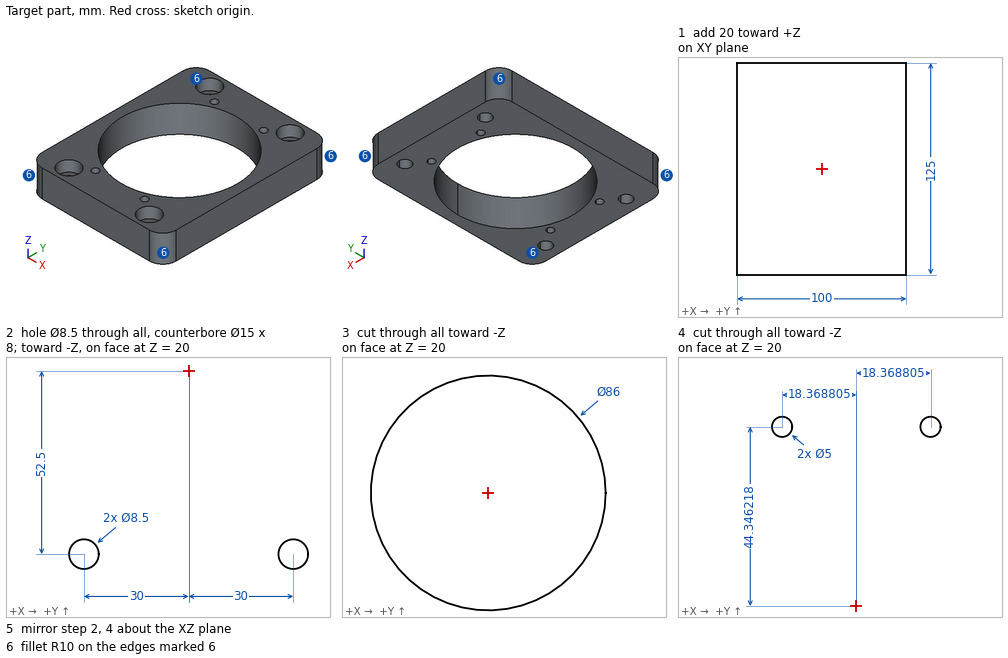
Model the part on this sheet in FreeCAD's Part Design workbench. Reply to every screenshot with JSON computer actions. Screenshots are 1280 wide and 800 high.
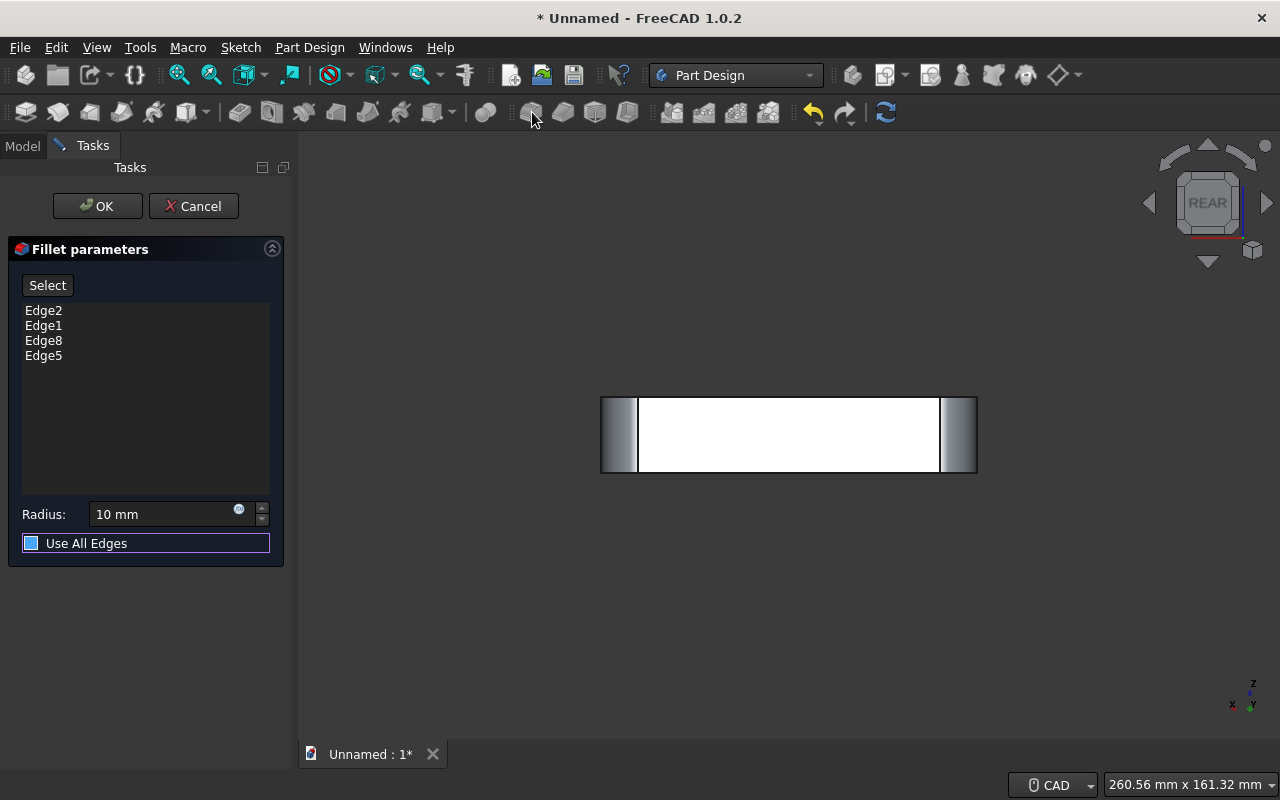
{"action": "left_click", "coordinate": [98, 206]}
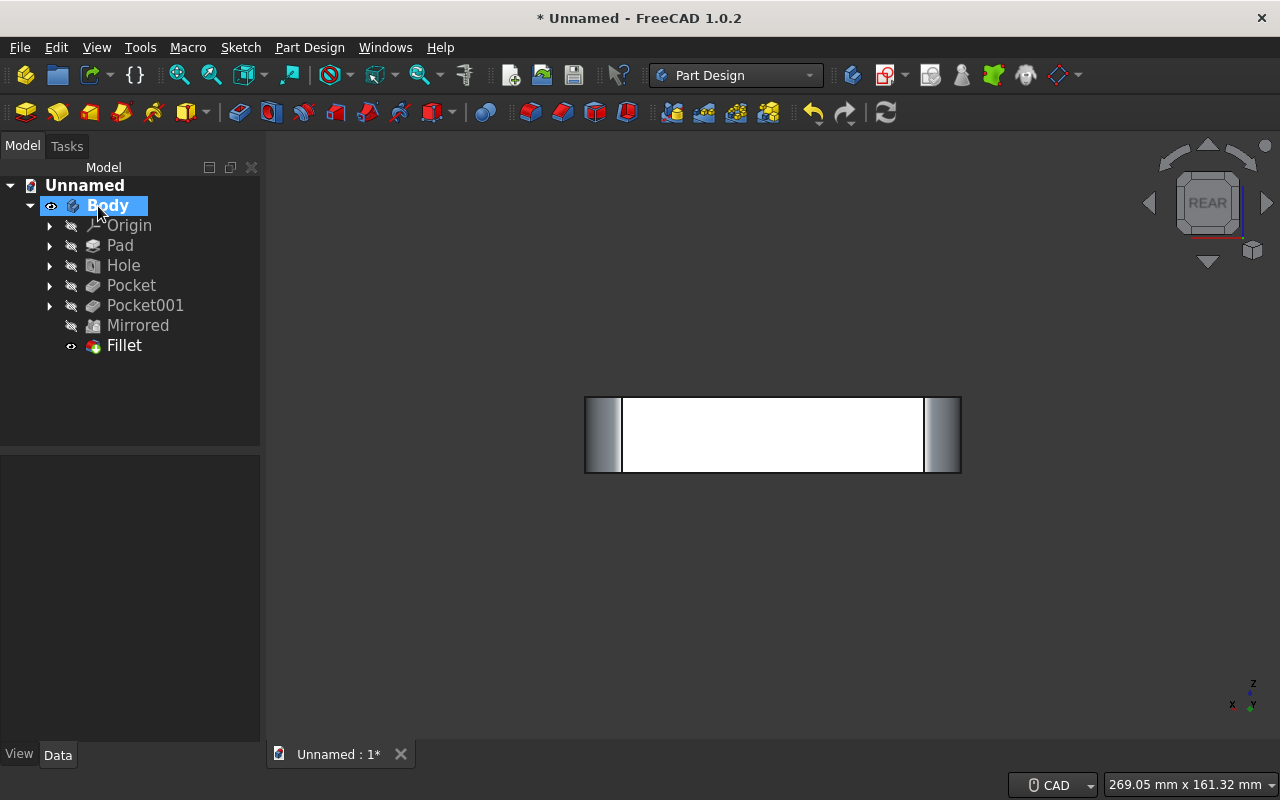
{"action": "key", "text": "0"}